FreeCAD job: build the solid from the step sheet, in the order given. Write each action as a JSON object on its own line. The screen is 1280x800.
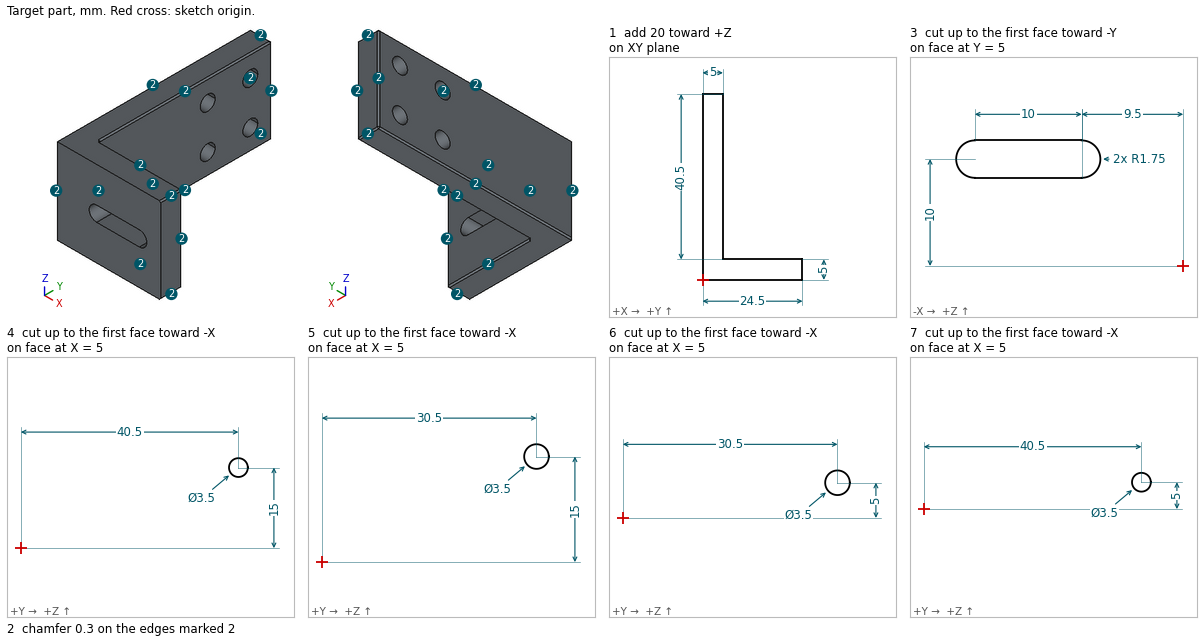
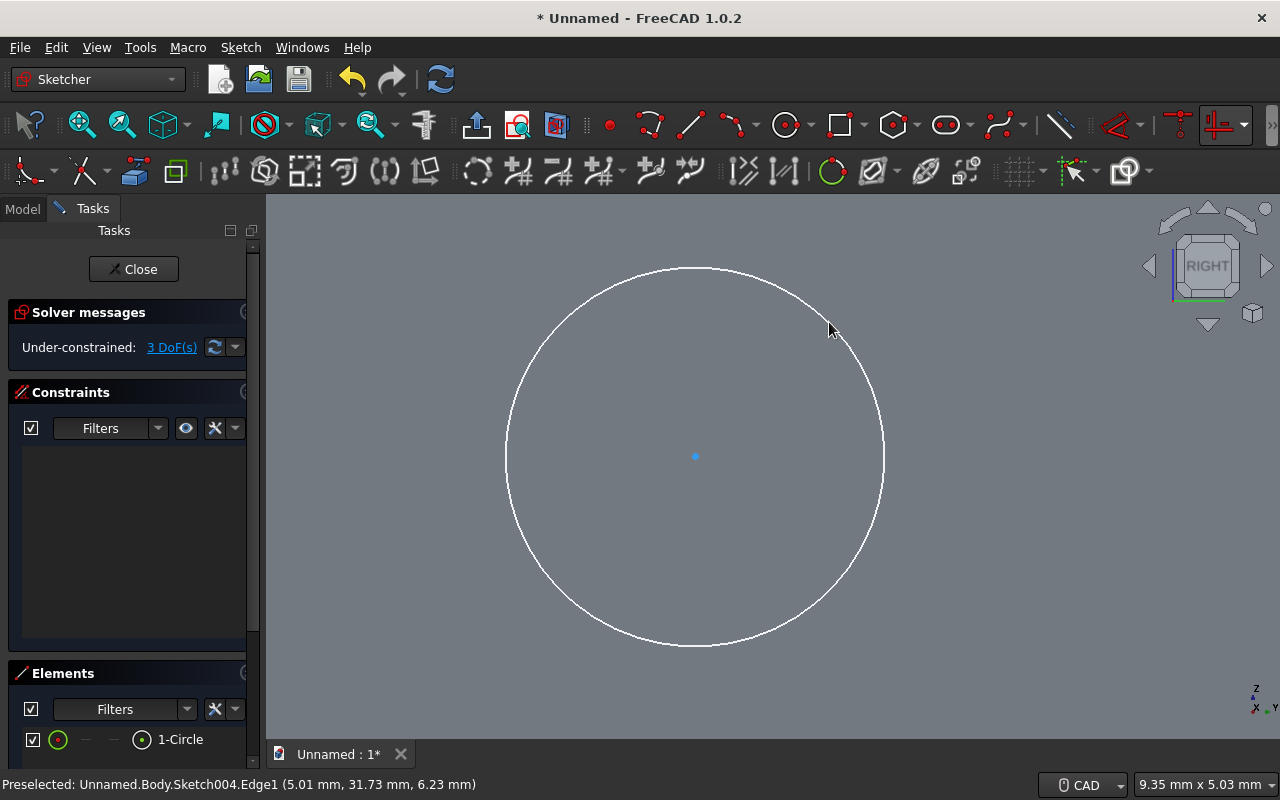
{"action": "left_click", "coordinate": [1116, 126]}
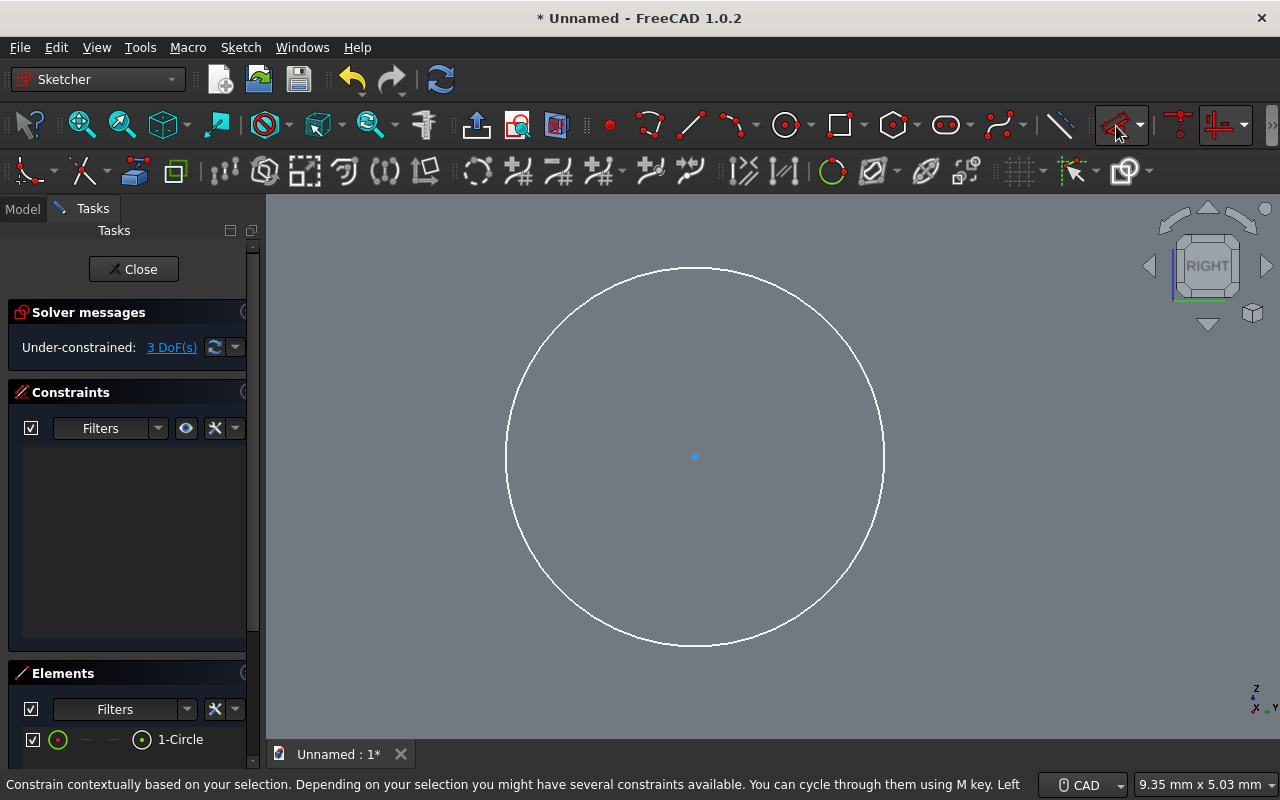
{"action": "left_click", "coordinate": [829, 323]}
{"action": "left_click", "coordinate": [852, 300]}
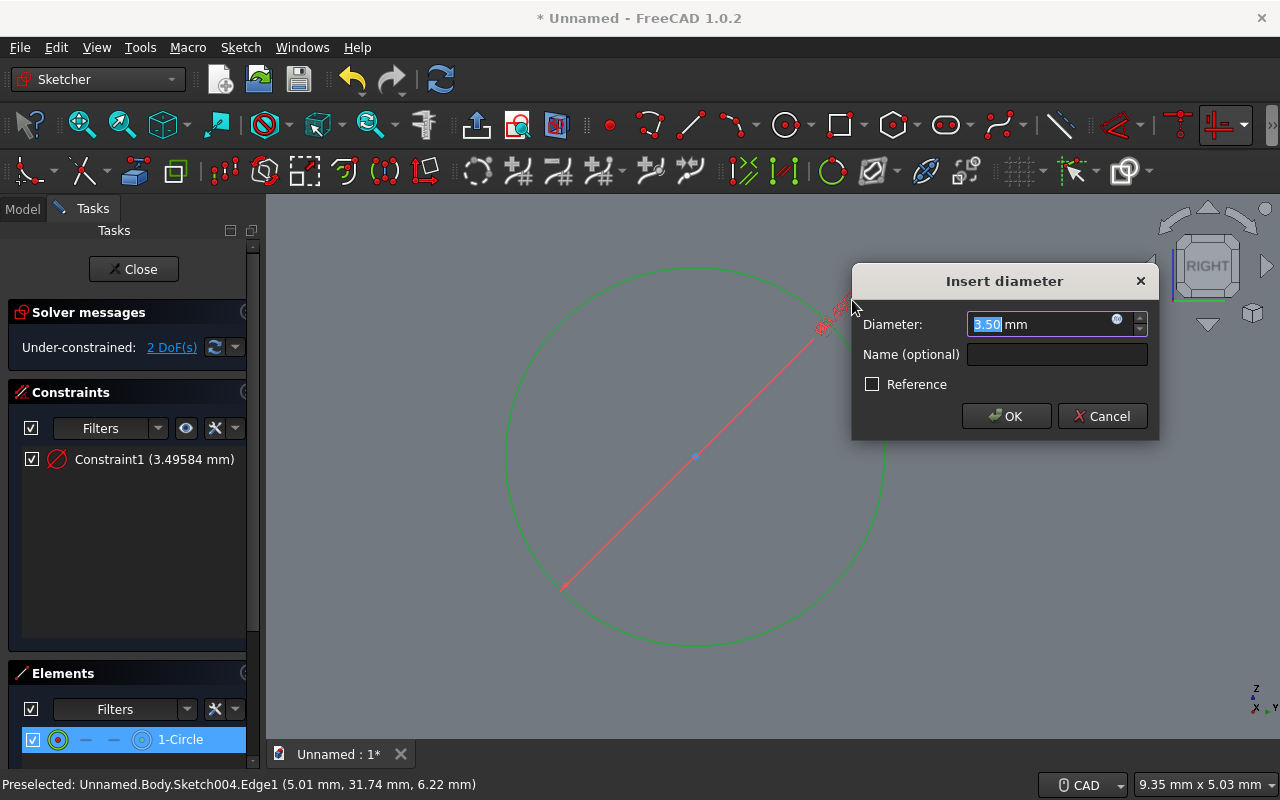
{"action": "type", "text": "3.5"}
{"action": "key", "text": "Return"}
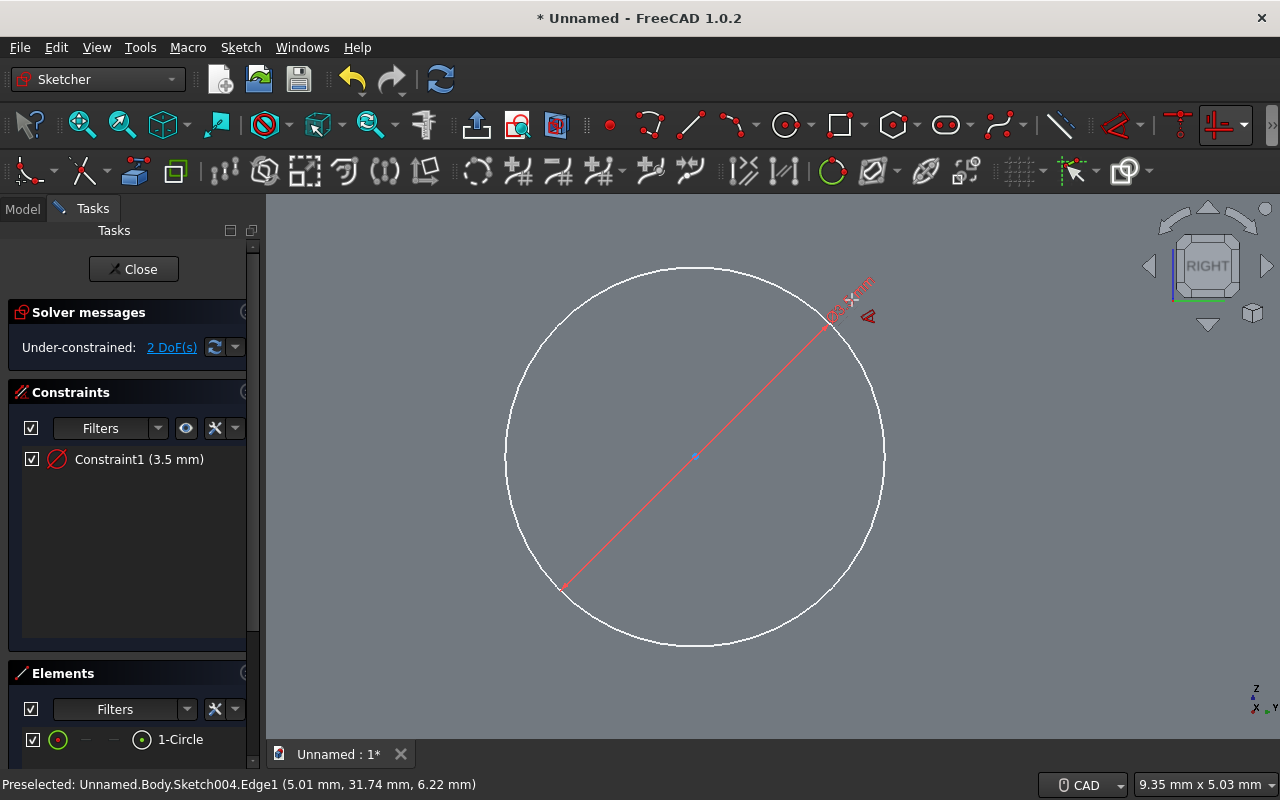
{"action": "left_click", "coordinate": [695, 457]}
{"action": "left_click", "coordinate": [729, 584]}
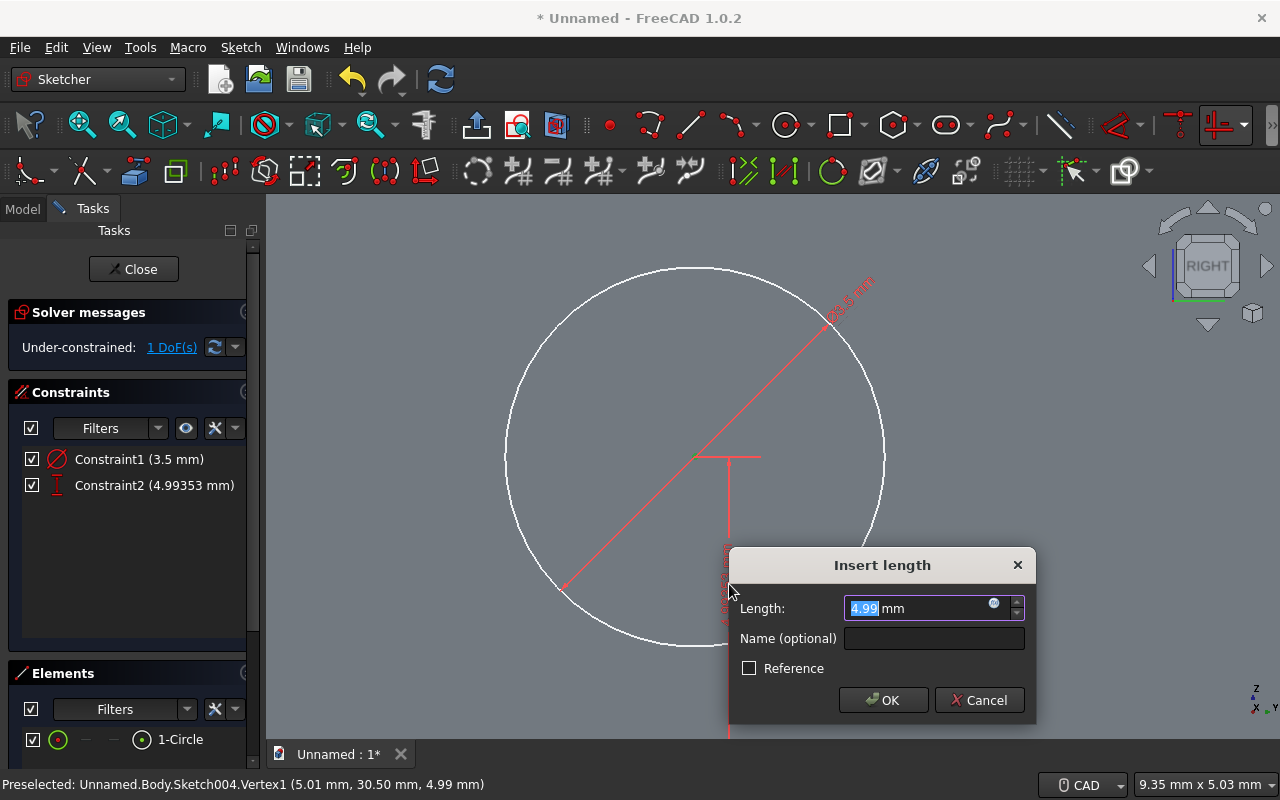
{"action": "type", "text": "5"}
{"action": "key", "text": "Return"}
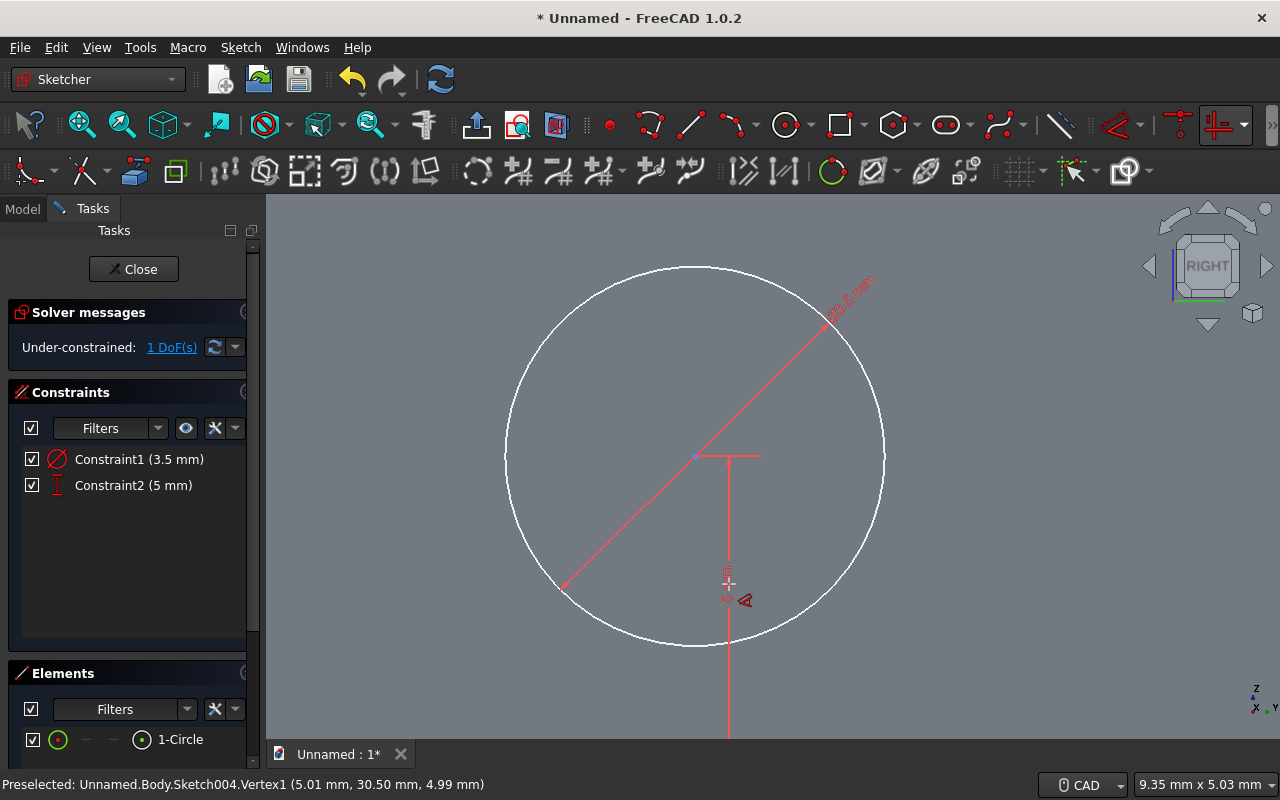
{"action": "left_click", "coordinate": [695, 456]}
{"action": "left_click", "coordinate": [494, 422]}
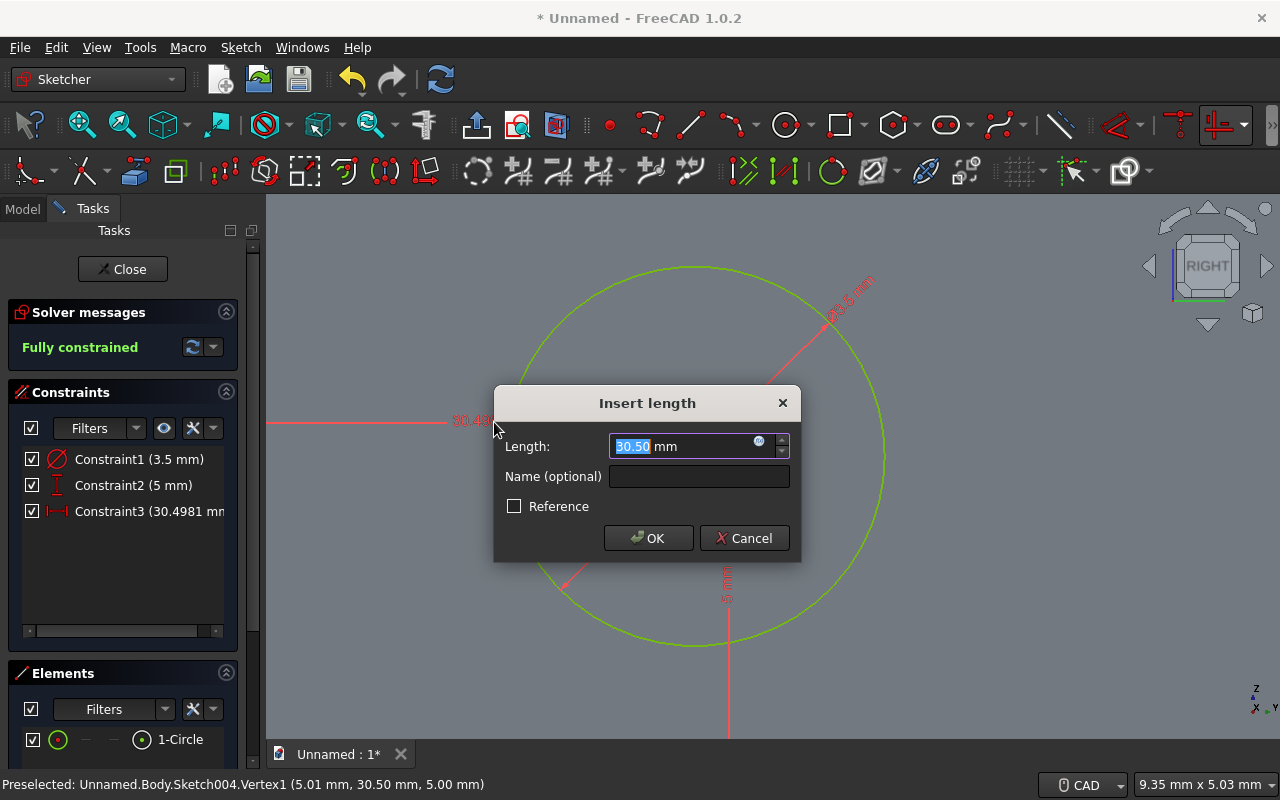
{"action": "type", "text": "30.5"}
{"action": "key", "text": "Return"}
{"action": "key", "text": "Escape"}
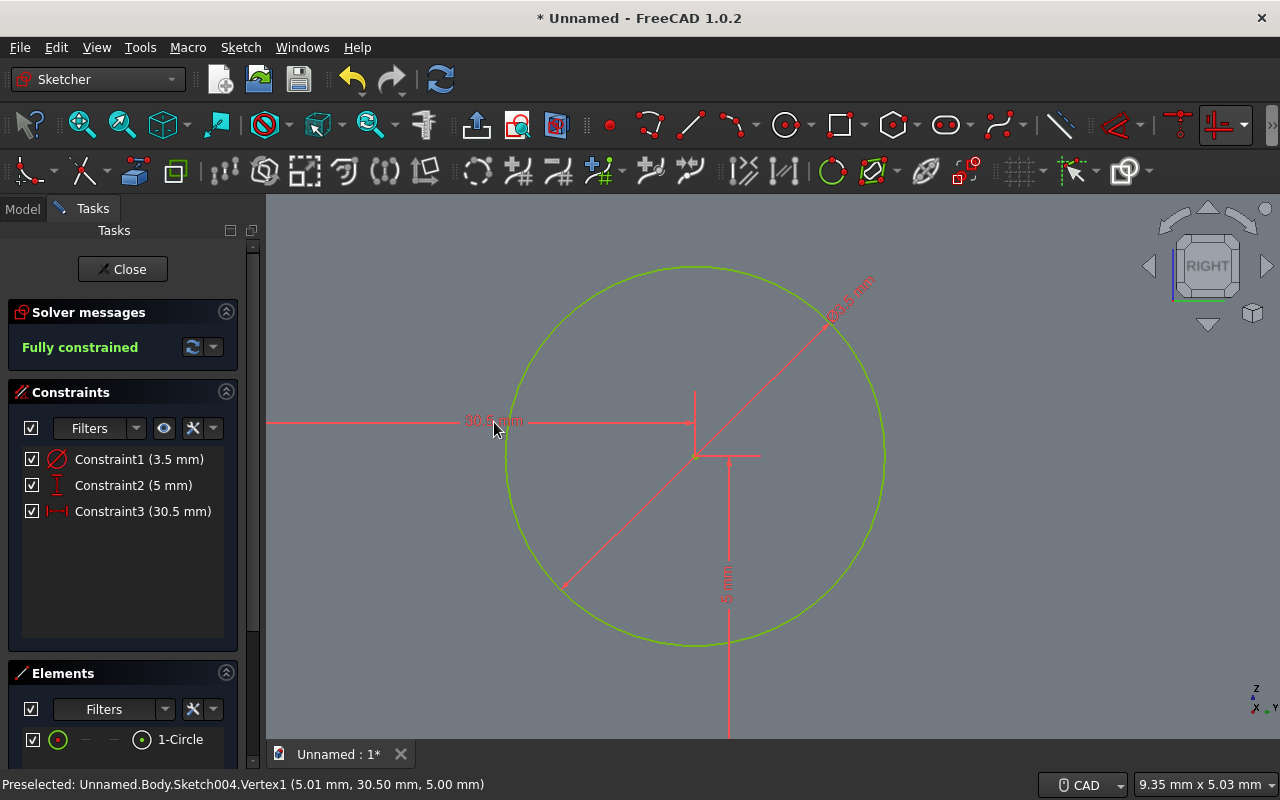
{"action": "left_click", "coordinate": [123, 269]}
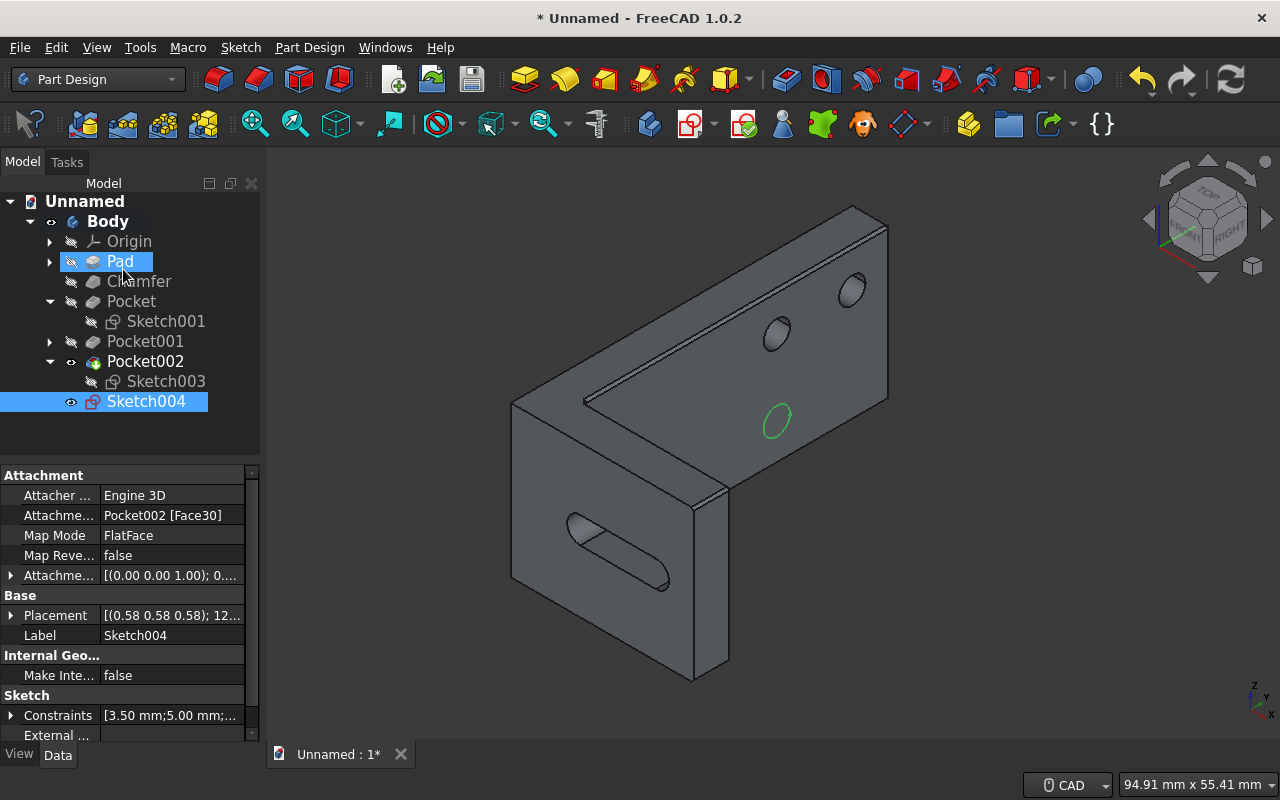
{"action": "left_click", "coordinate": [788, 80]}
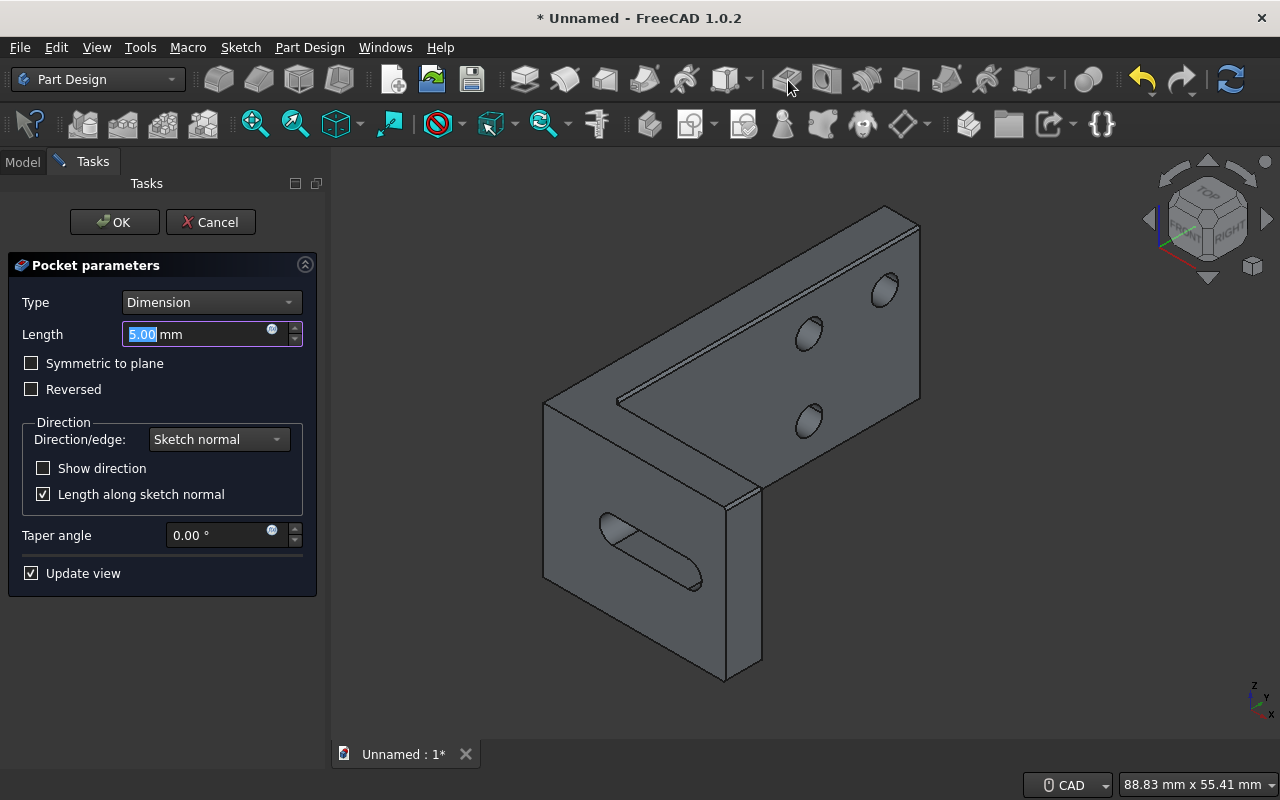
{"action": "left_click", "coordinate": [212, 302]}